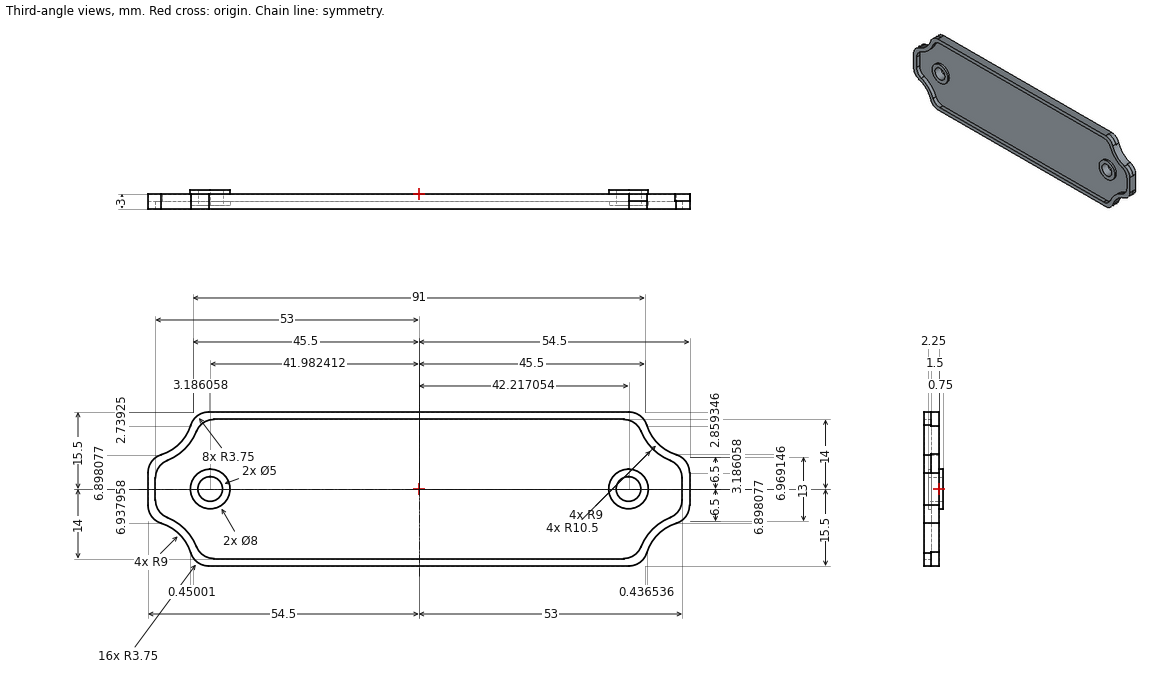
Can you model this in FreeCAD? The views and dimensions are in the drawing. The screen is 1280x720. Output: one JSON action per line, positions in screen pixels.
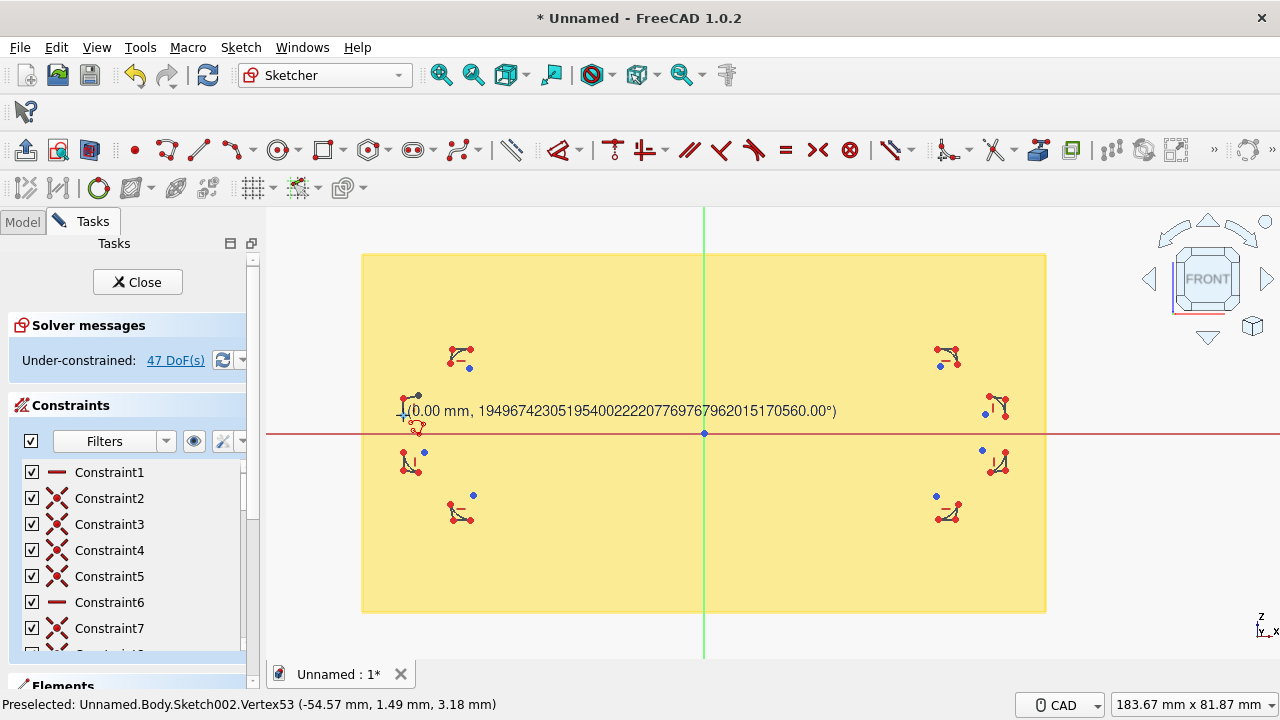
{"action": "left_click", "coordinate": [232, 150]}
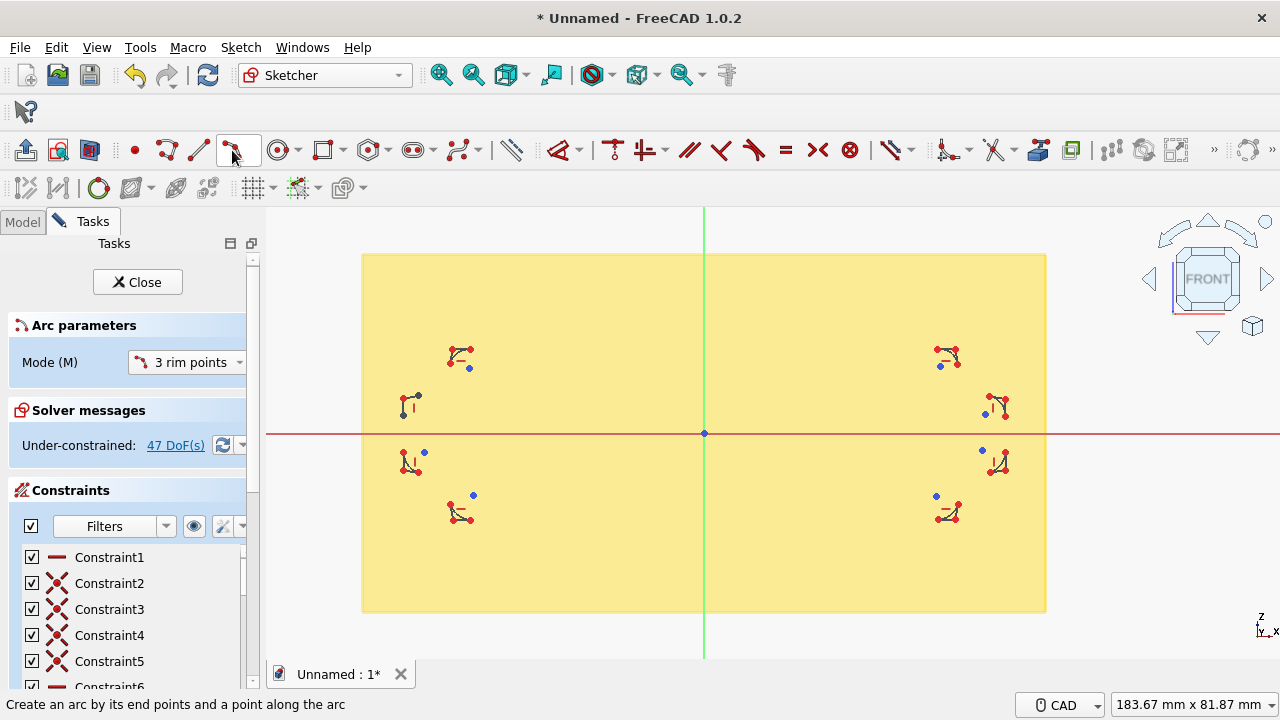
{"action": "scroll", "coordinate": [403, 415], "scroll_direction": "up", "scroll_amount": 3}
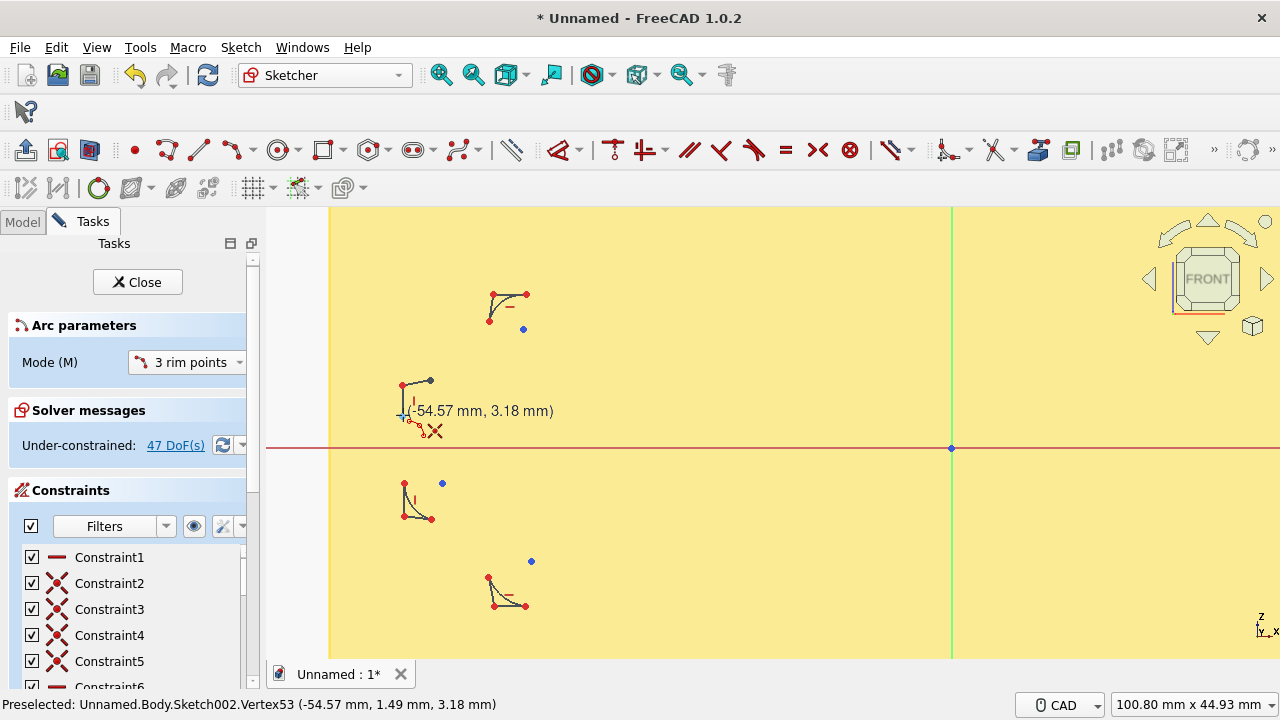
{"action": "left_click", "coordinate": [403, 416]}
{"action": "left_click", "coordinate": [430, 380]}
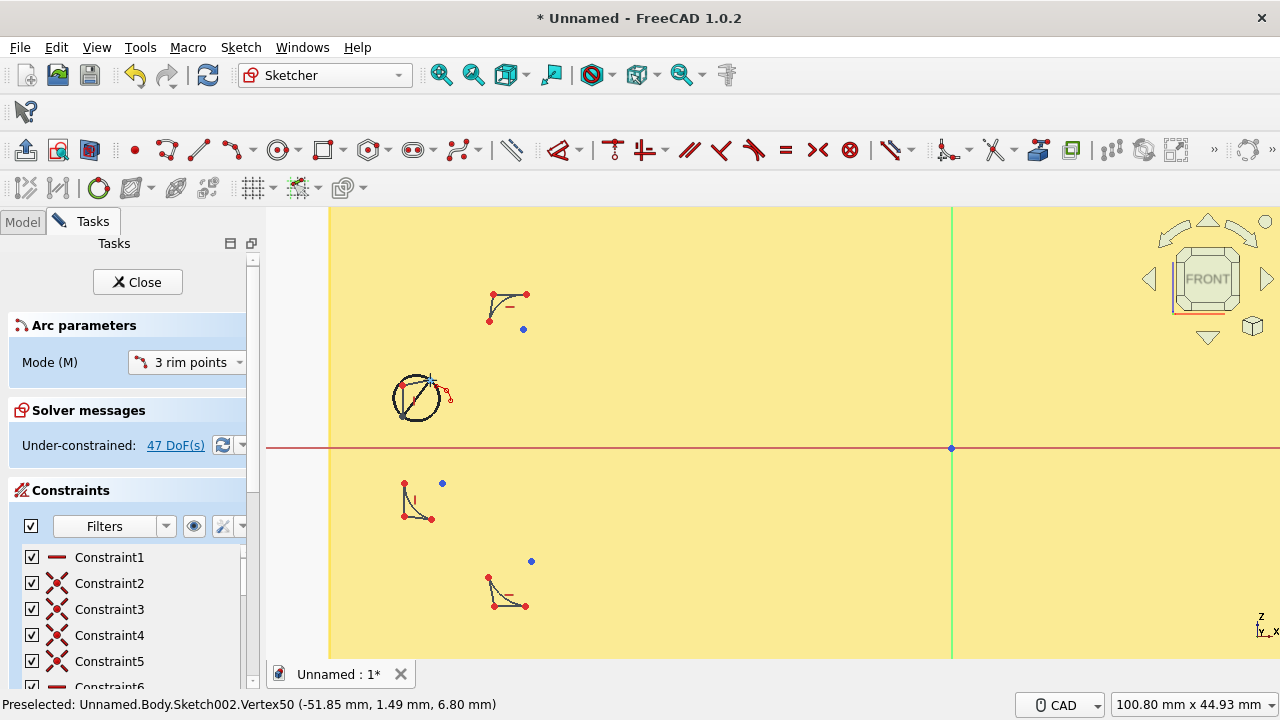
{"action": "scroll", "coordinate": [411, 393], "scroll_direction": "up", "scroll_amount": 4}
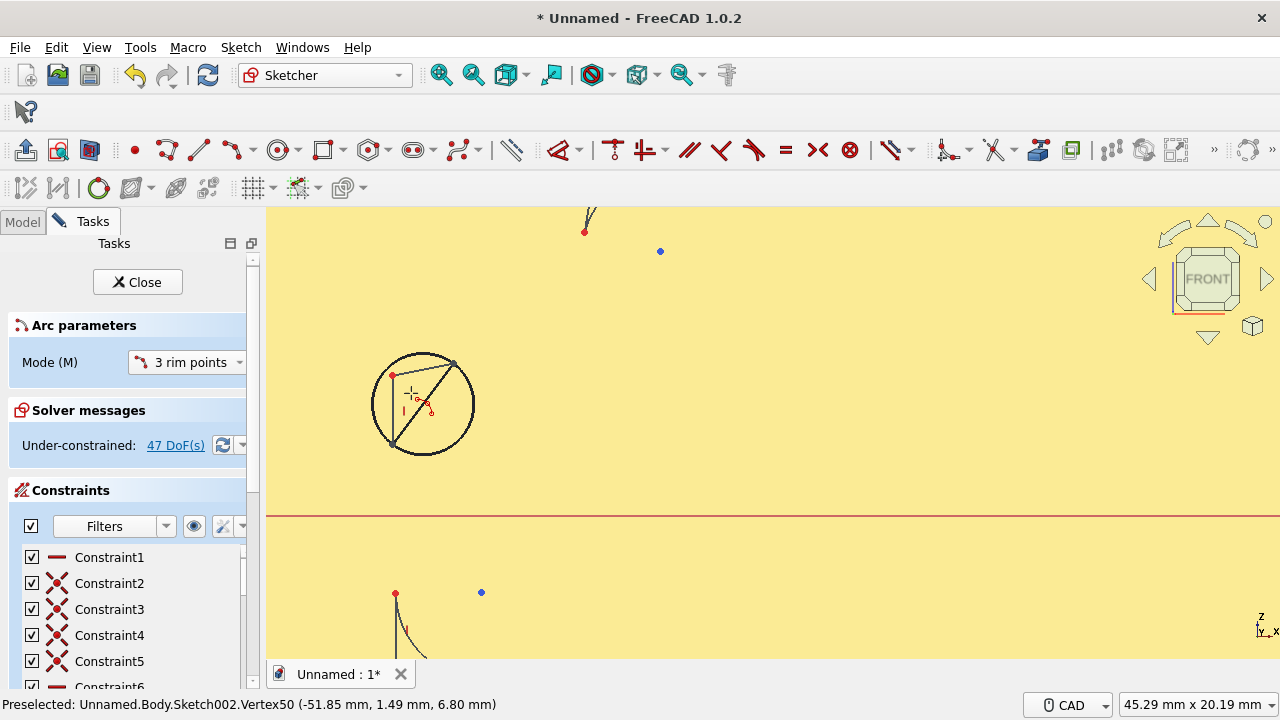
{"action": "left_click", "coordinate": [411, 392]}
{"action": "key", "text": "Escape"}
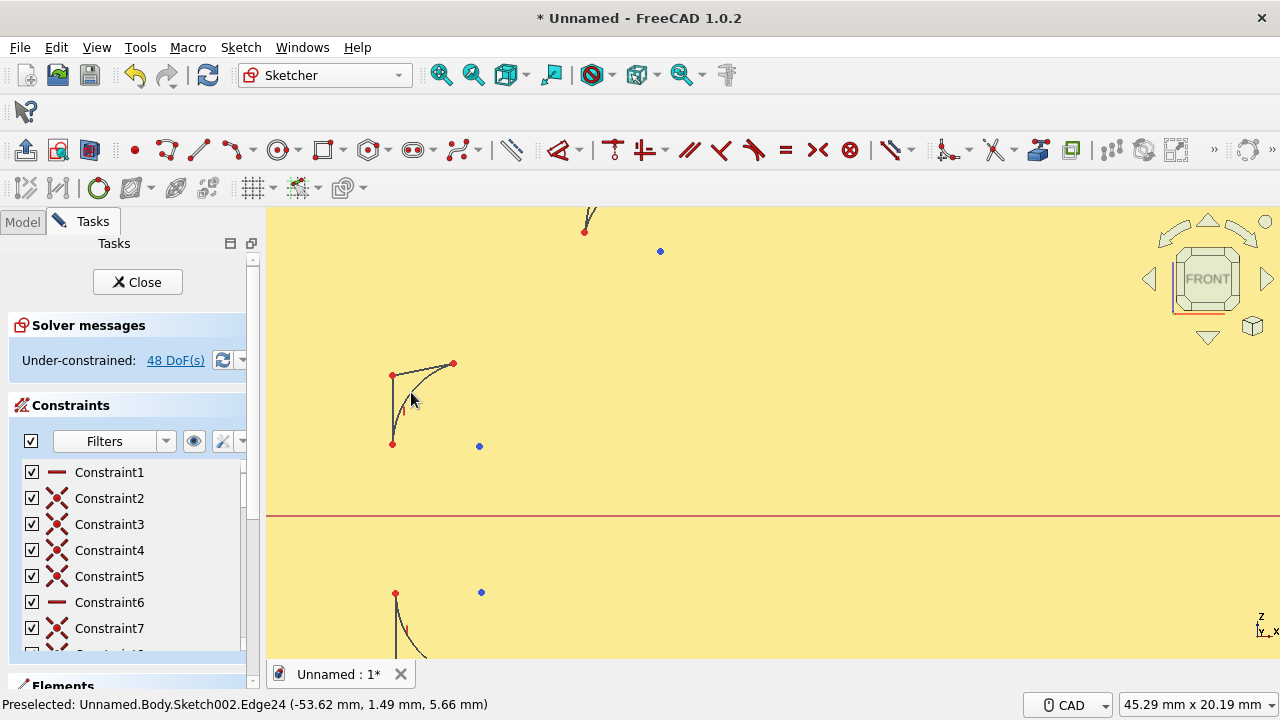
{"action": "scroll", "coordinate": [407, 406], "scroll_direction": "down", "scroll_amount": 7}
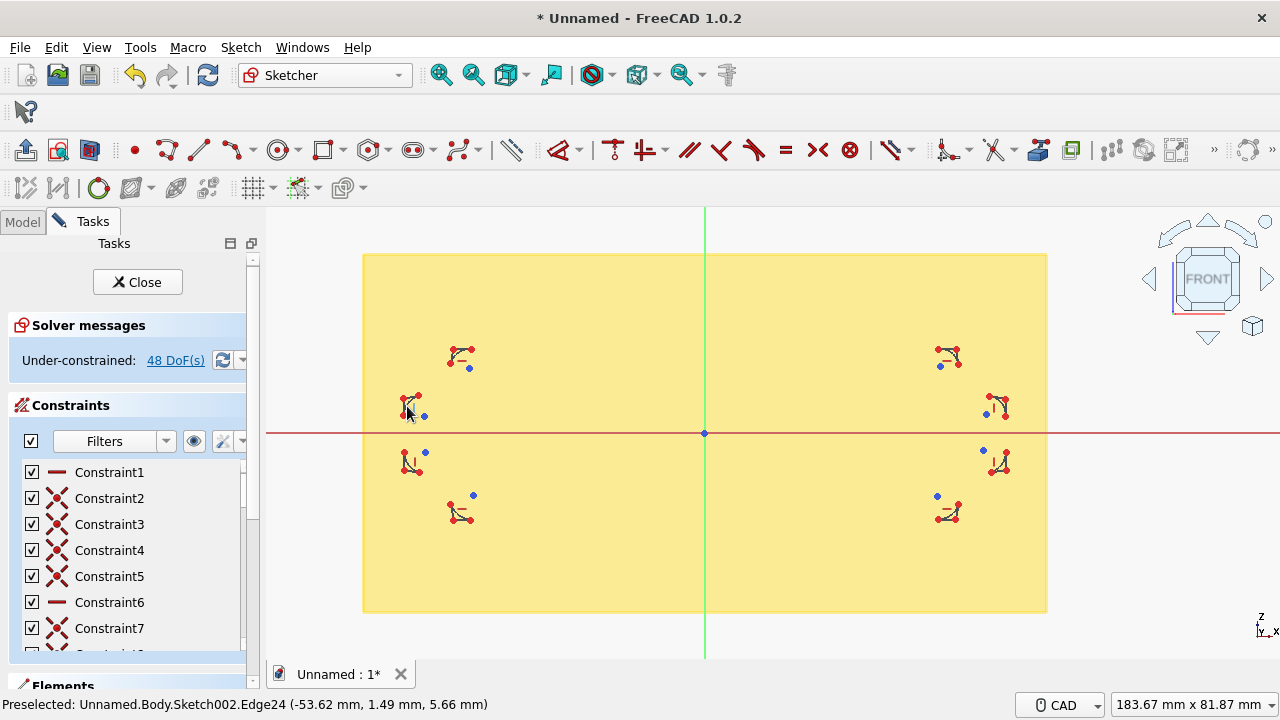
{"action": "scroll", "coordinate": [459, 349], "scroll_direction": "up", "scroll_amount": 9}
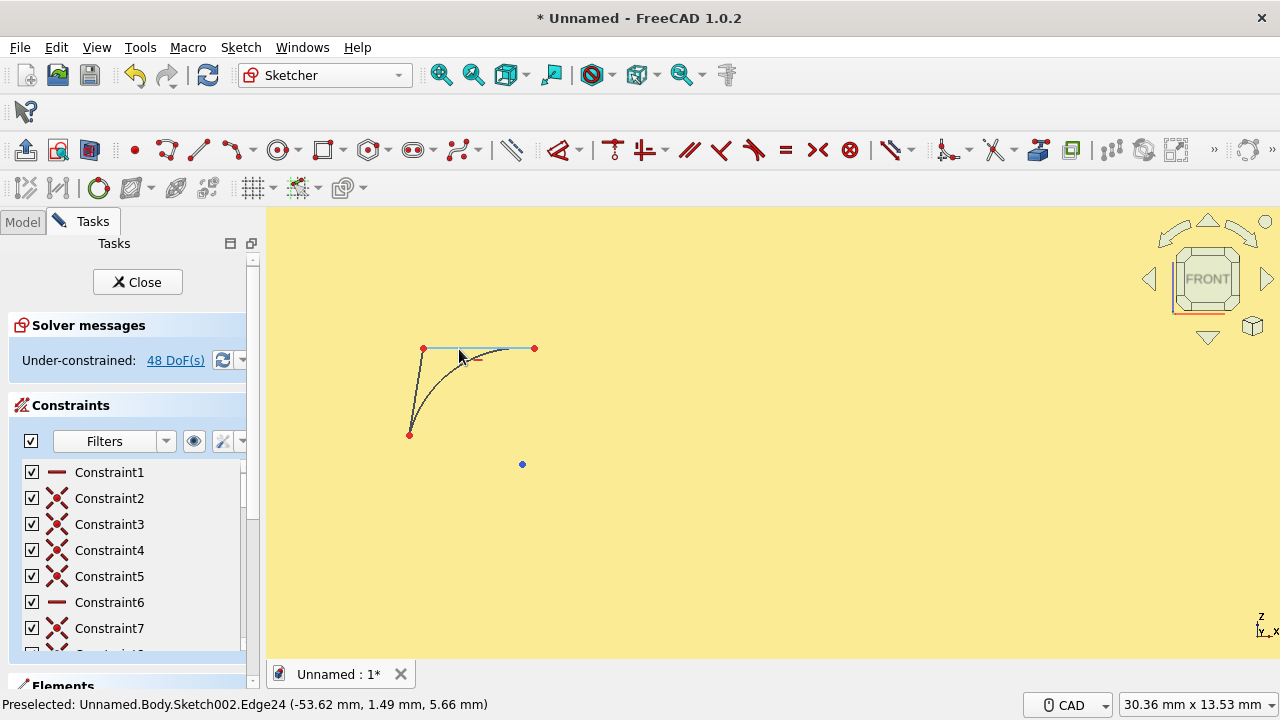
{"action": "left_click", "coordinate": [457, 348]}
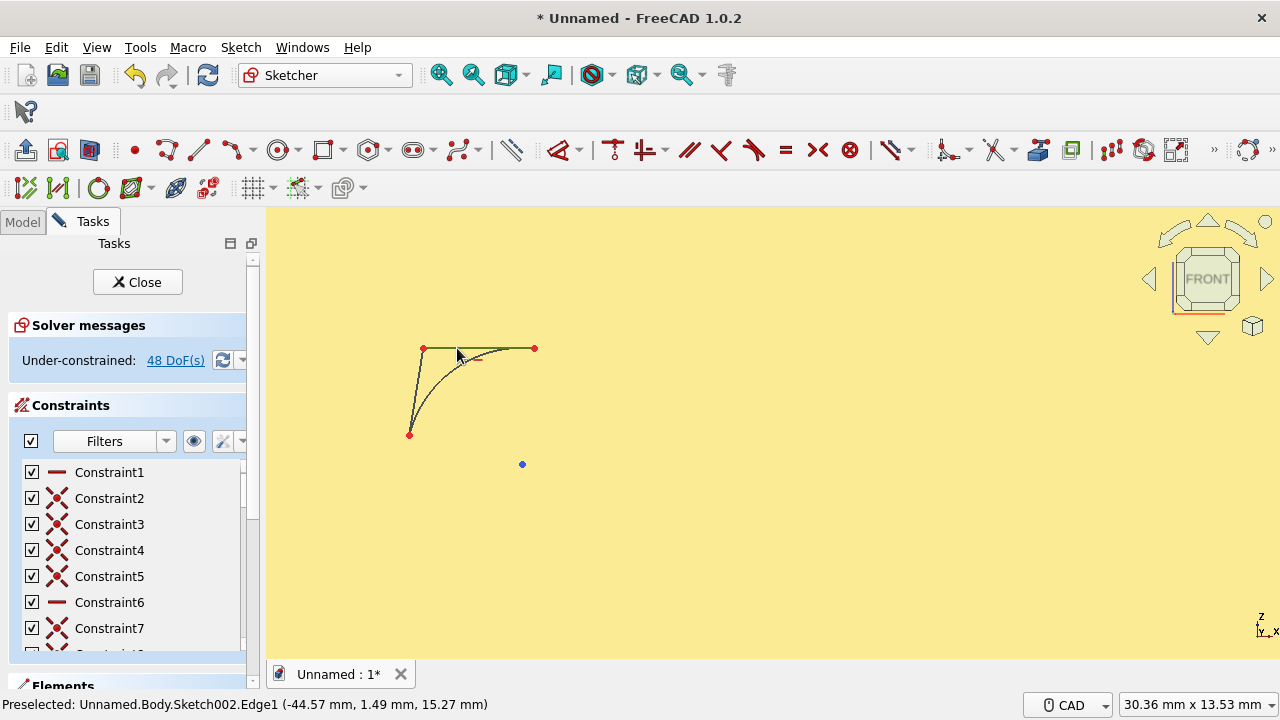
{"action": "left_click", "coordinate": [431, 391]}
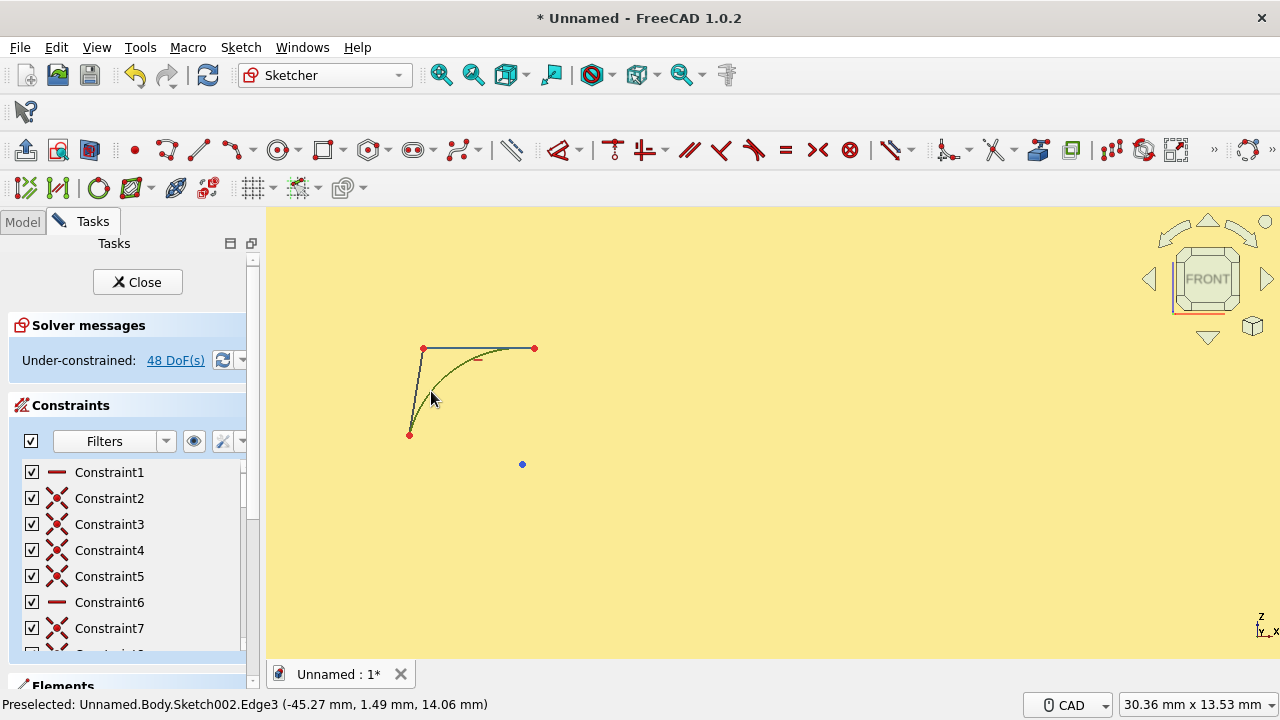
{"action": "left_click", "coordinate": [754, 150]}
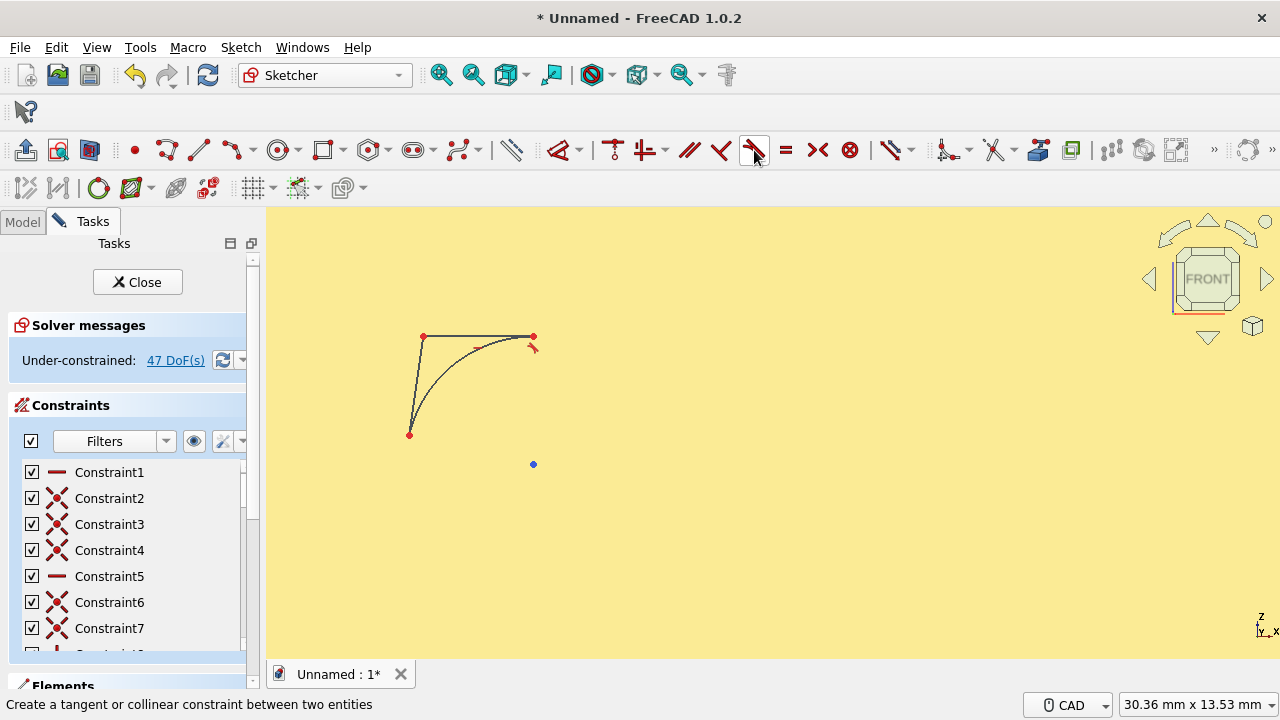
{"action": "scroll", "coordinate": [459, 349], "scroll_direction": "down", "scroll_amount": 9}